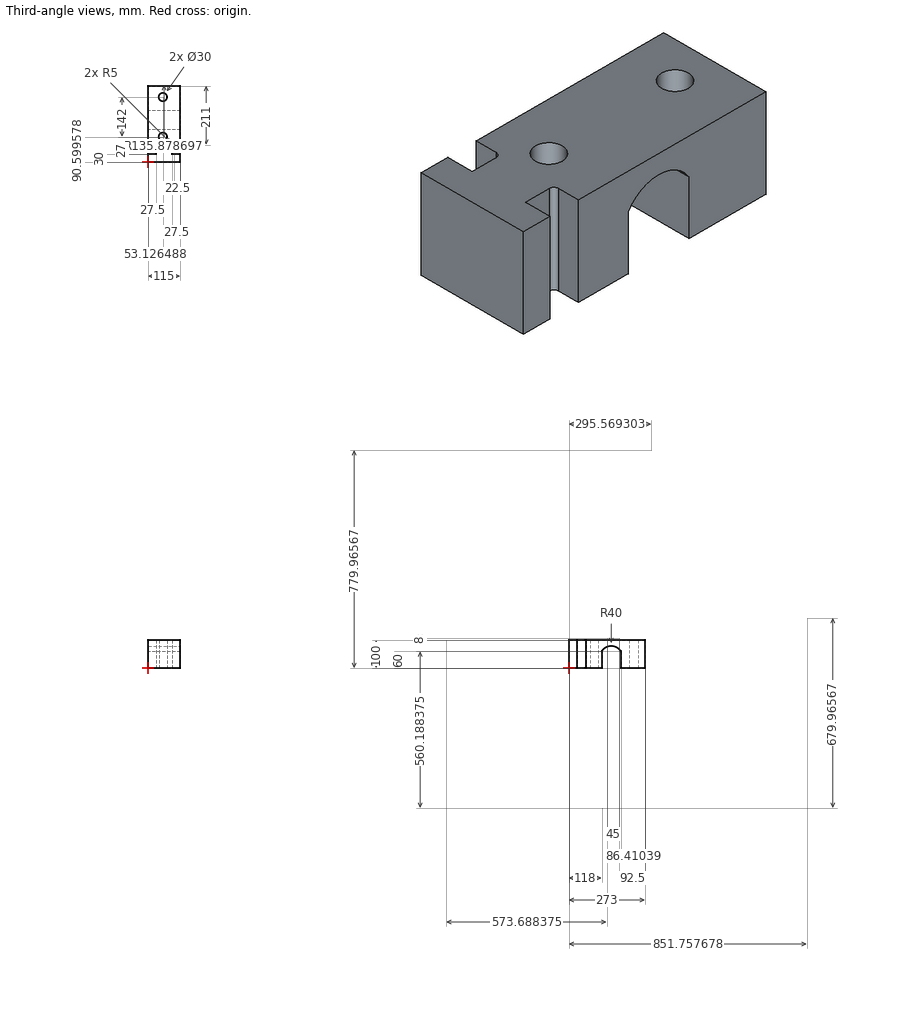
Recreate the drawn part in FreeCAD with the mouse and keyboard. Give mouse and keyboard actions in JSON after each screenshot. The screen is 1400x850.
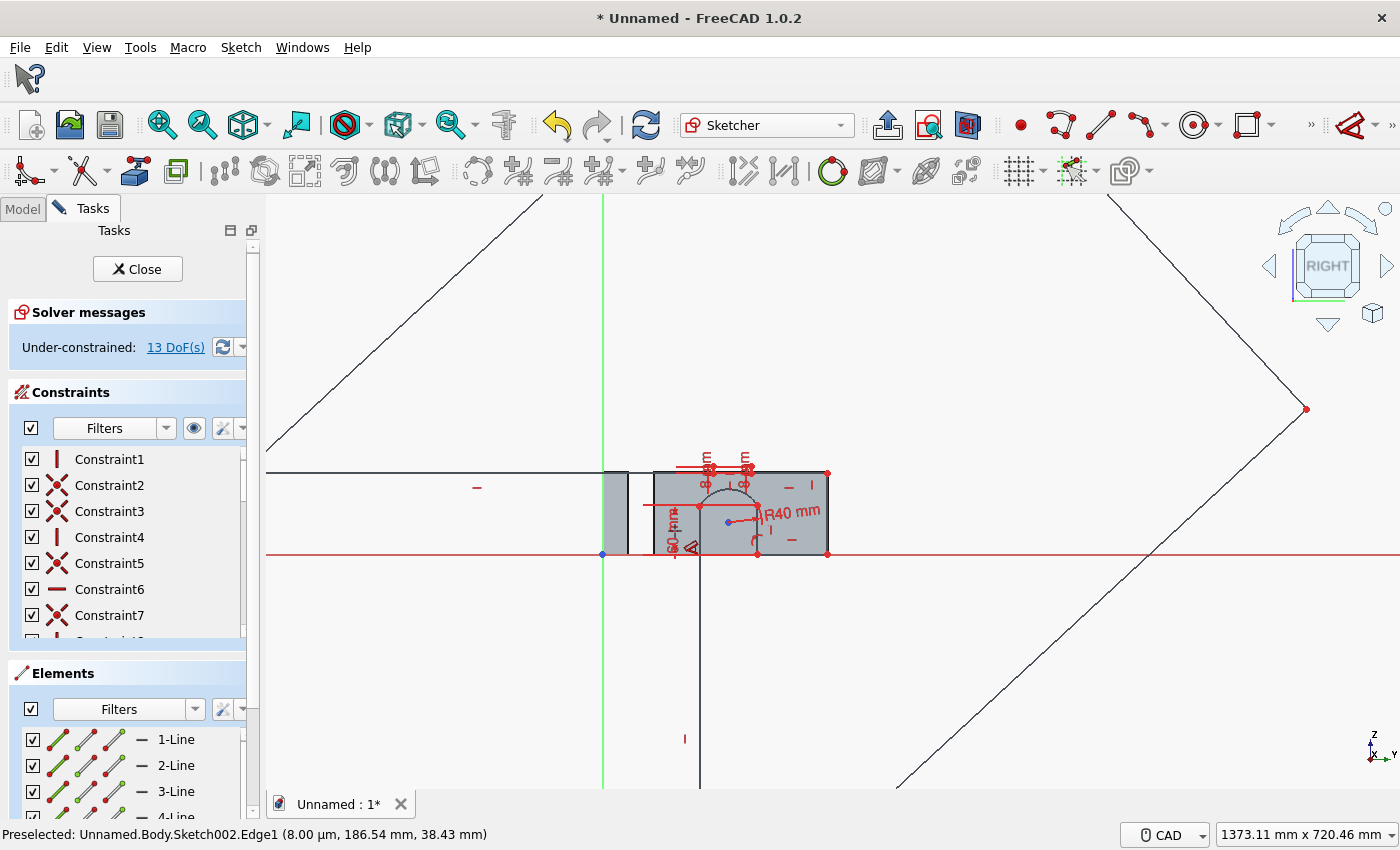
{"action": "left_click", "coordinate": [740, 467]}
{"action": "left_click", "coordinate": [733, 433]}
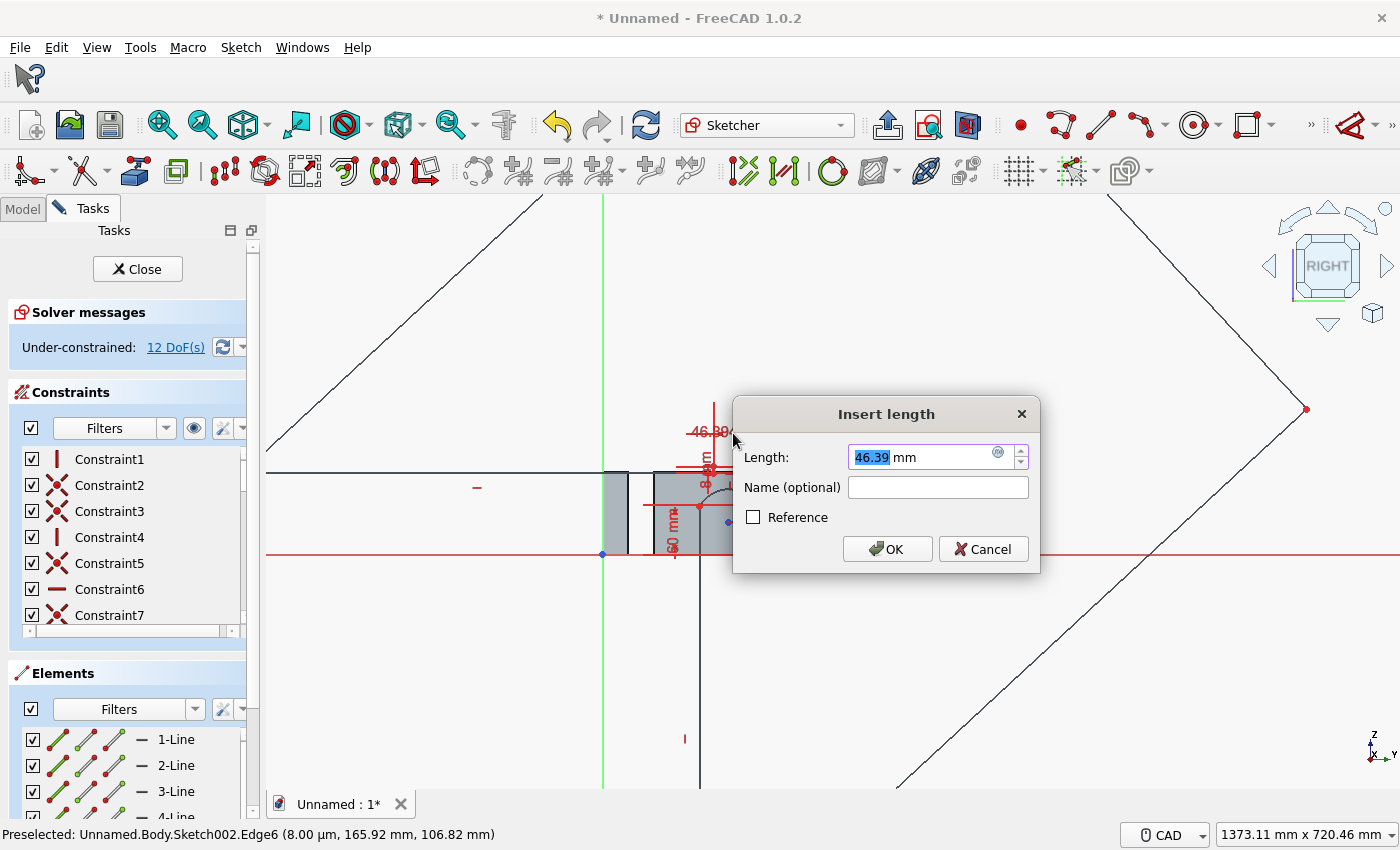
{"action": "type", "text": "45"}
{"action": "key", "text": "Return"}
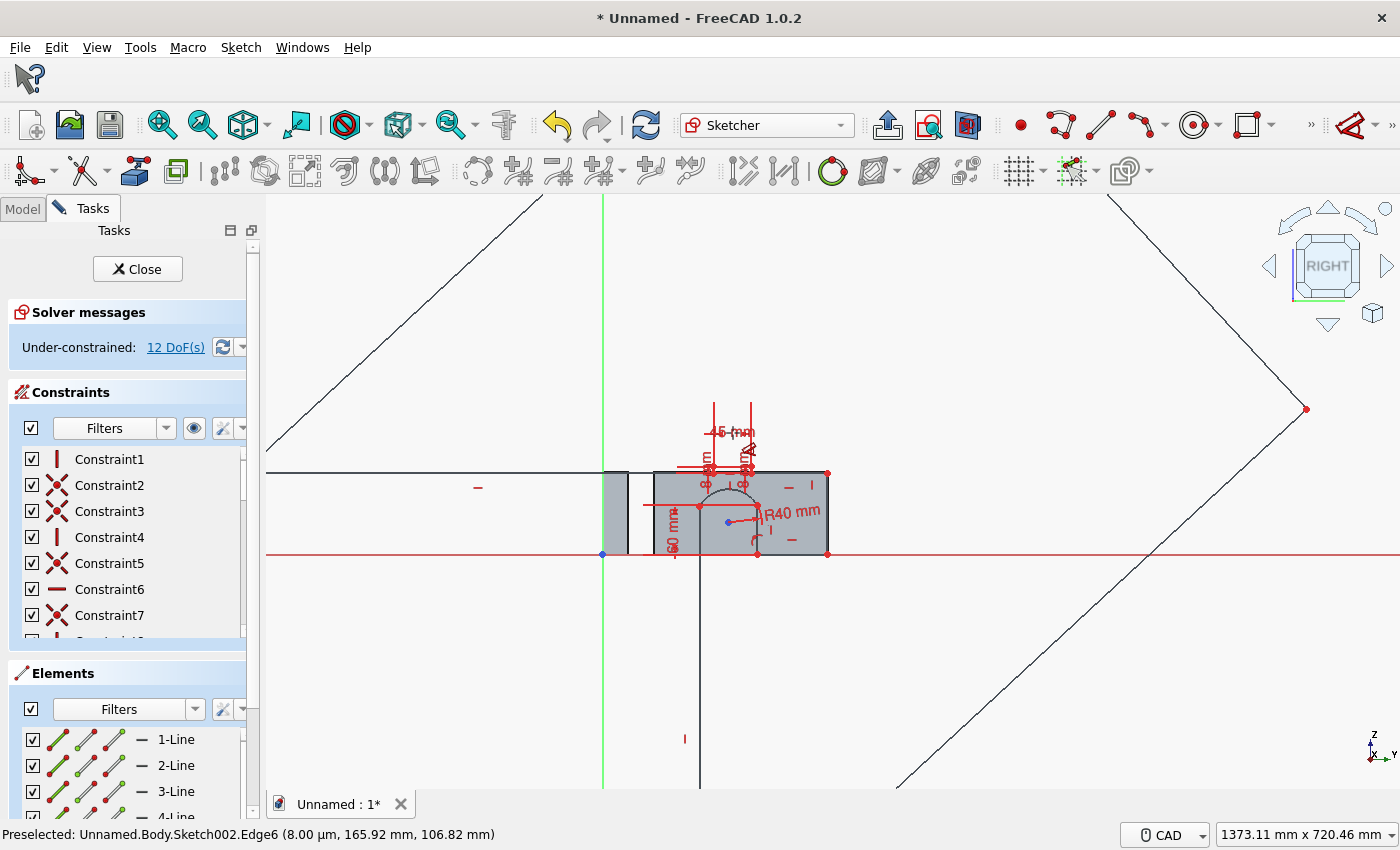
{"action": "left_click", "coordinate": [827, 530]}
{"action": "left_click", "coordinate": [861, 485]}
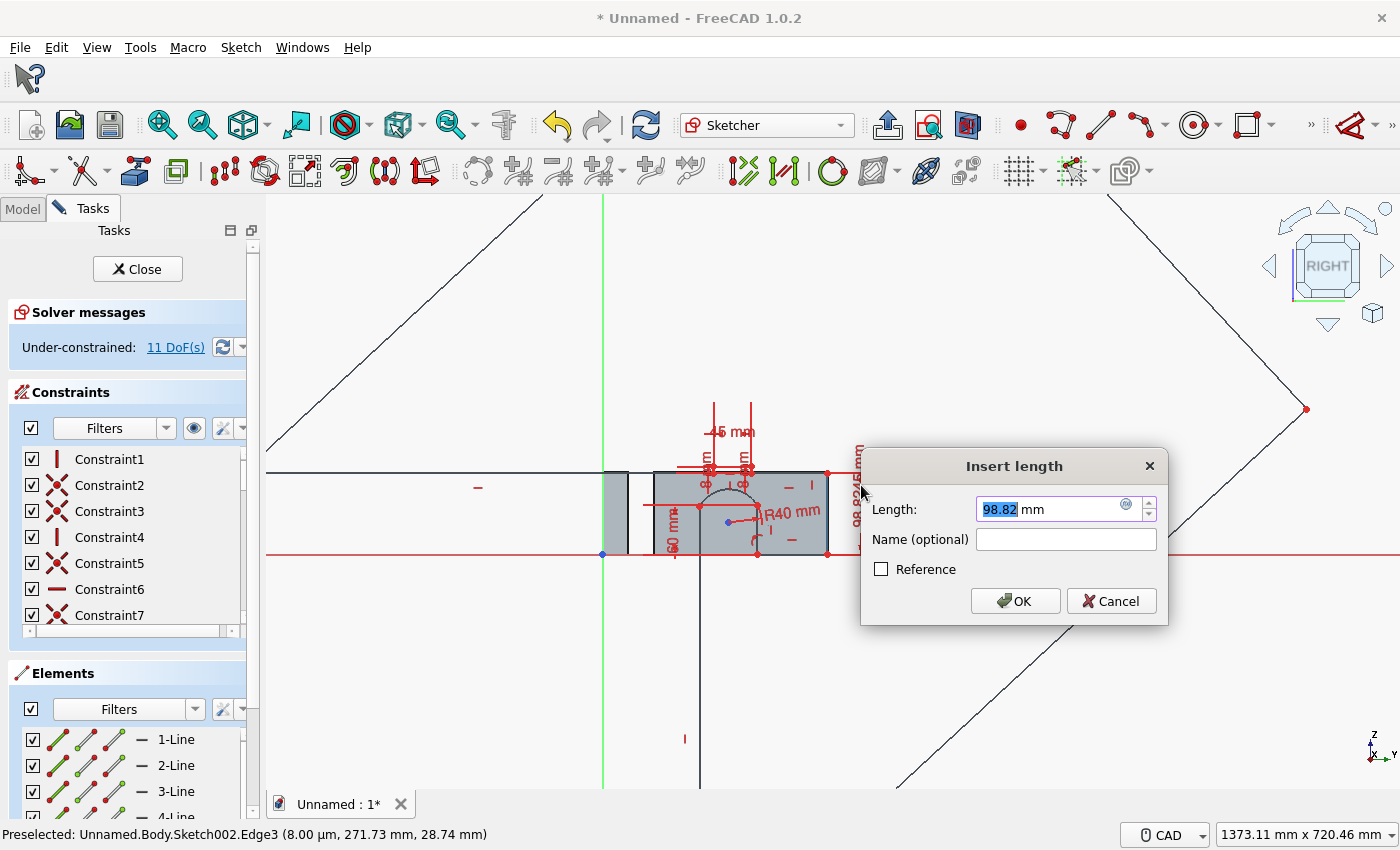
{"action": "type", "text": "100"}
{"action": "key", "text": "Return"}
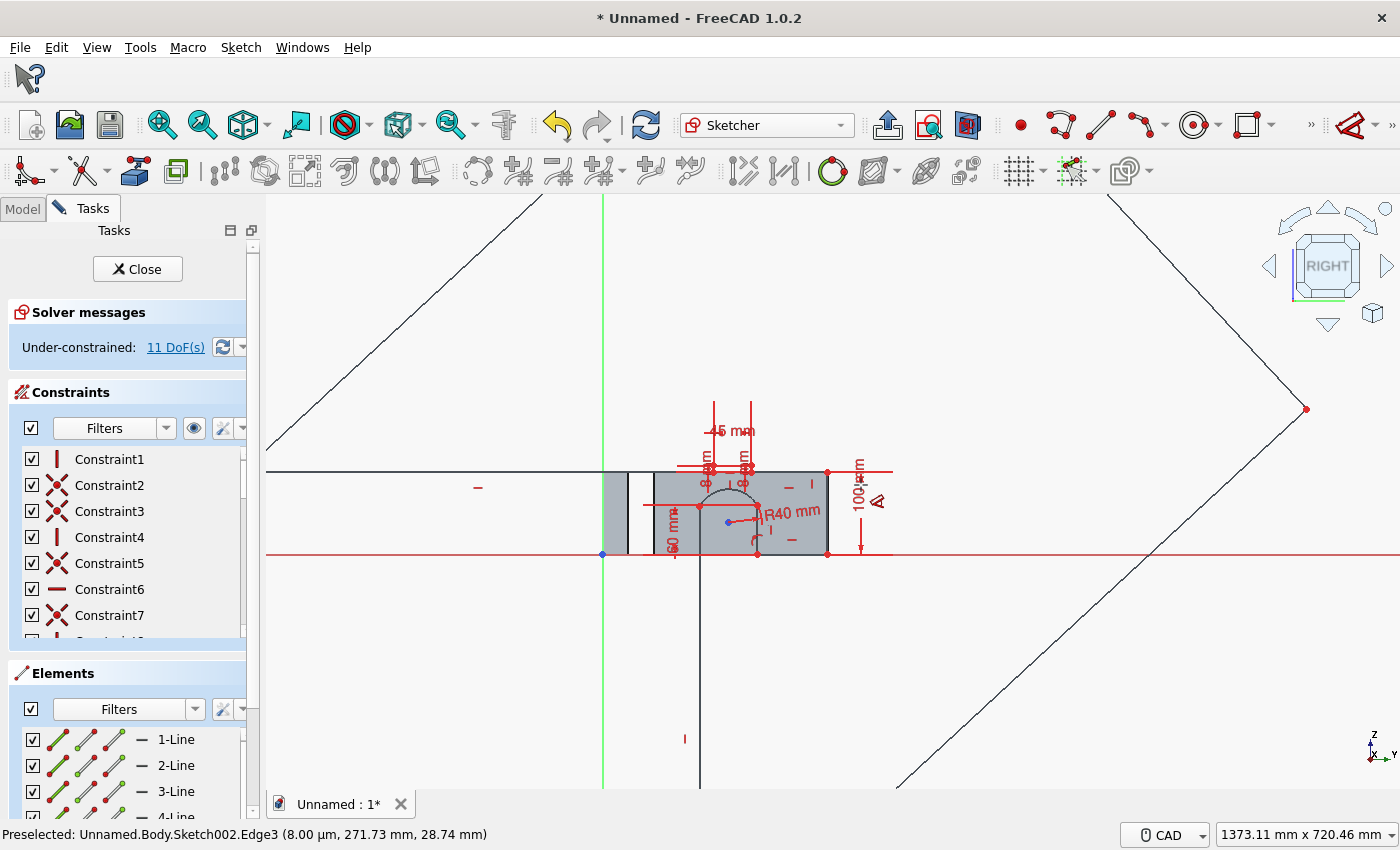
{"action": "left_click", "coordinate": [700, 506]}
{"action": "left_click", "coordinate": [569, 530]}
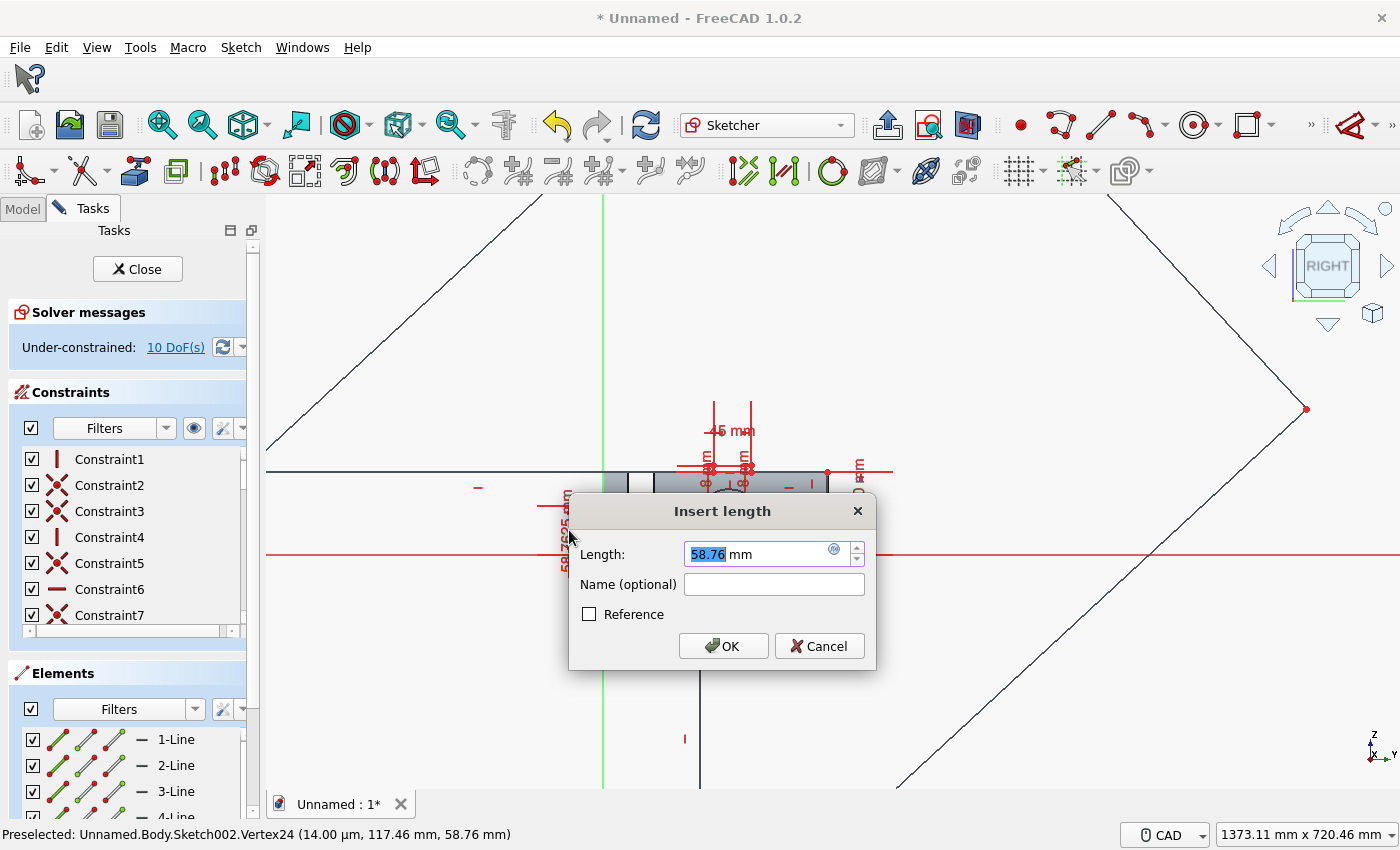
{"action": "type", "text": "60"}
{"action": "key", "text": "Return"}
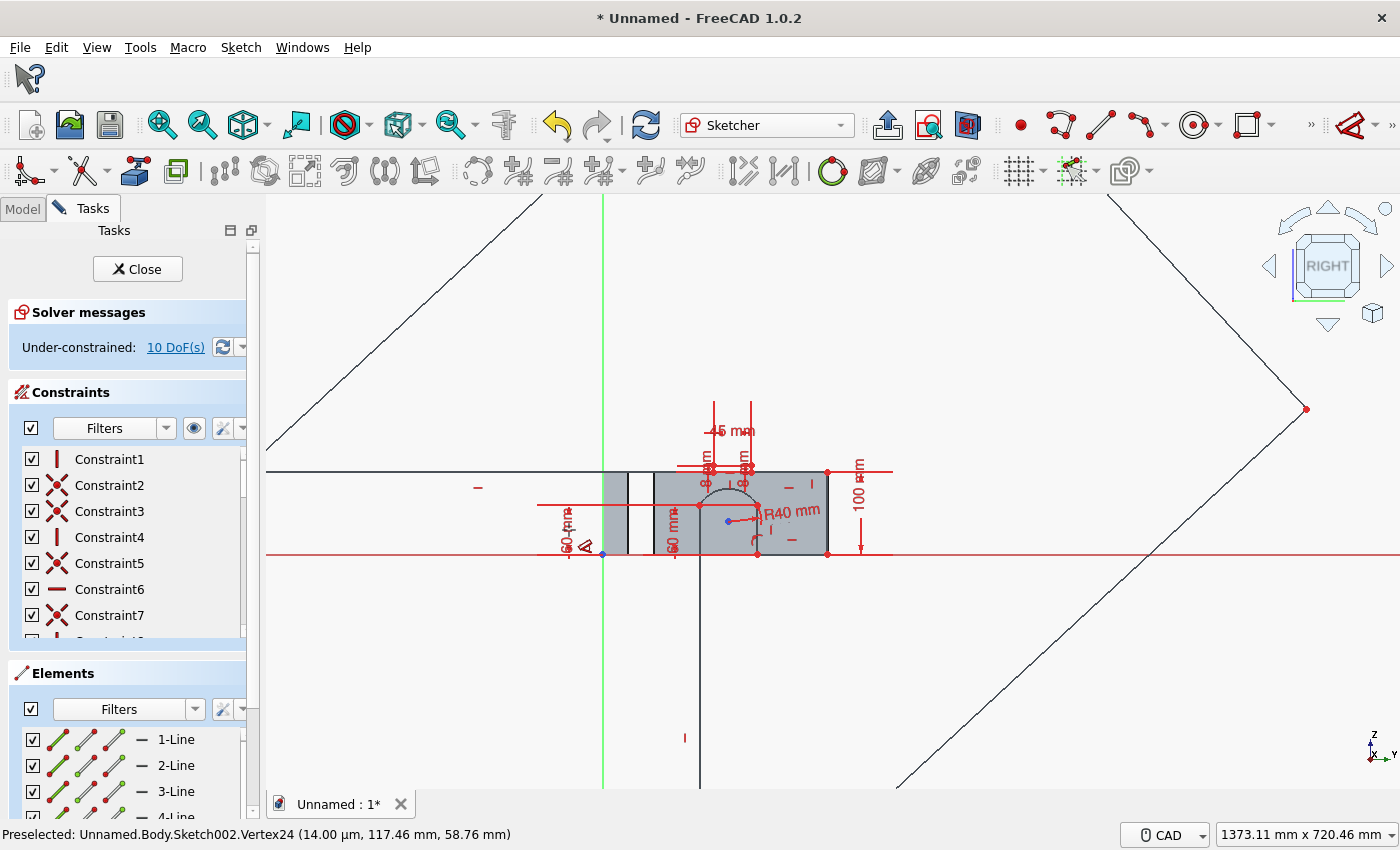
{"action": "left_click", "coordinate": [804, 472]}
{"action": "left_click", "coordinate": [807, 438]}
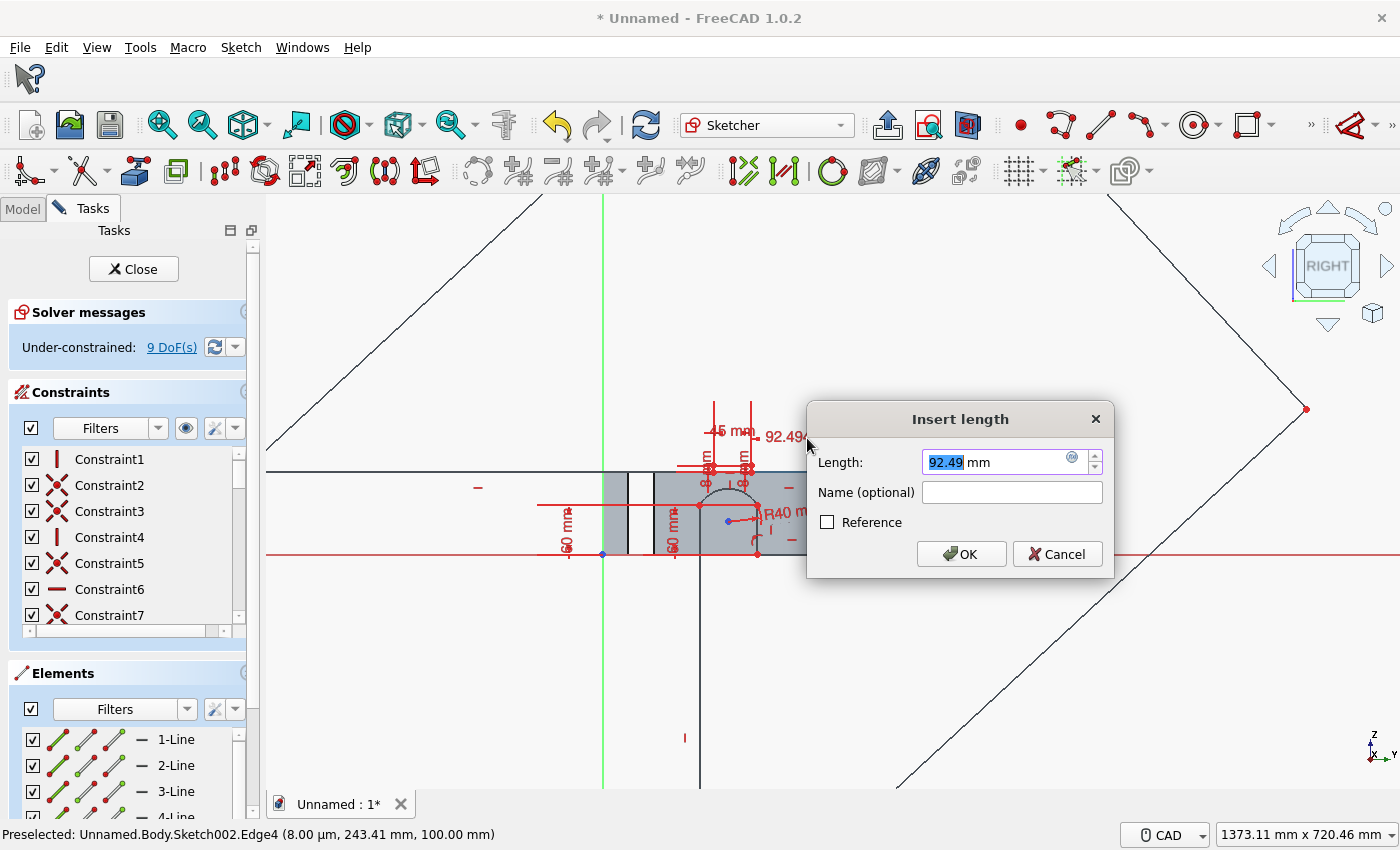
{"action": "type", "text": "92.5"}
{"action": "key", "text": "Return"}